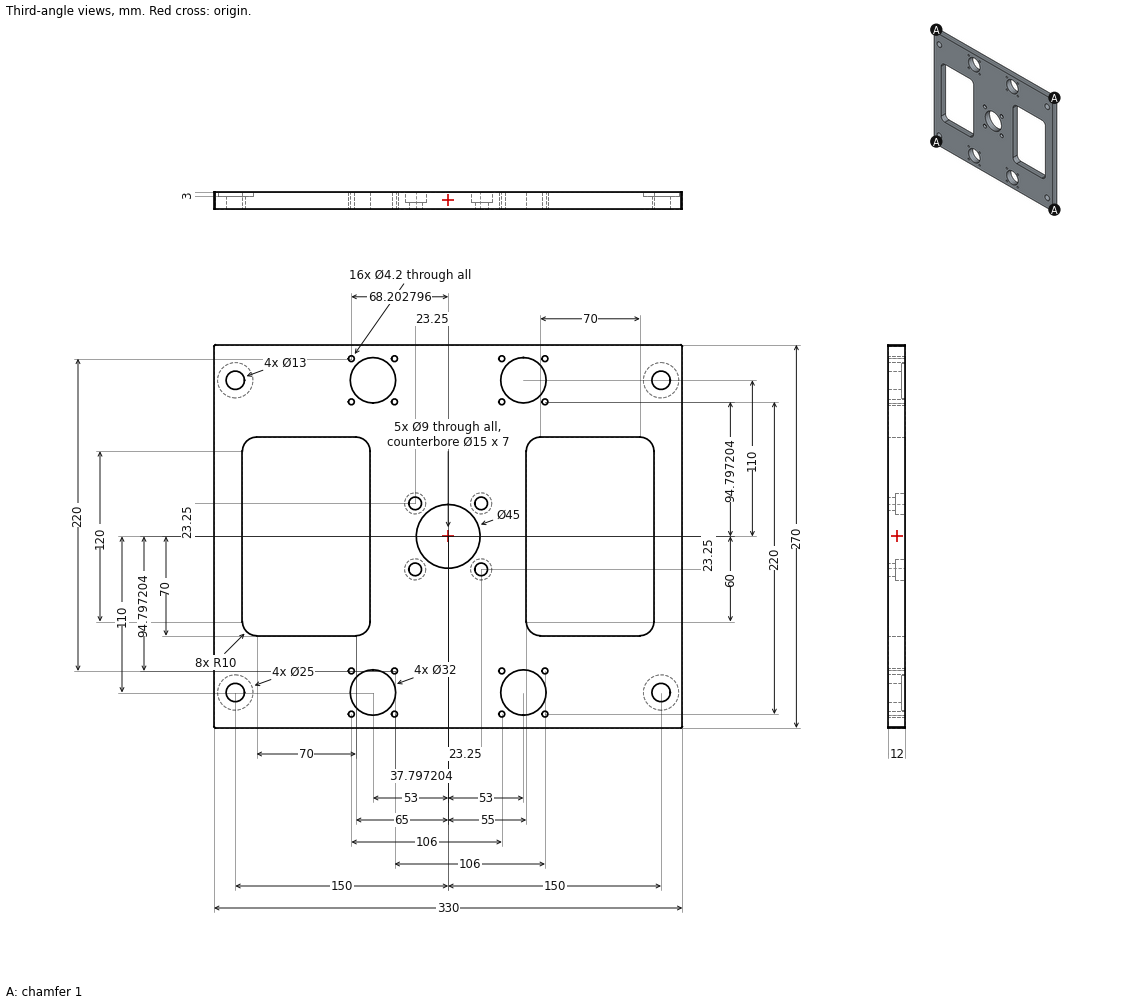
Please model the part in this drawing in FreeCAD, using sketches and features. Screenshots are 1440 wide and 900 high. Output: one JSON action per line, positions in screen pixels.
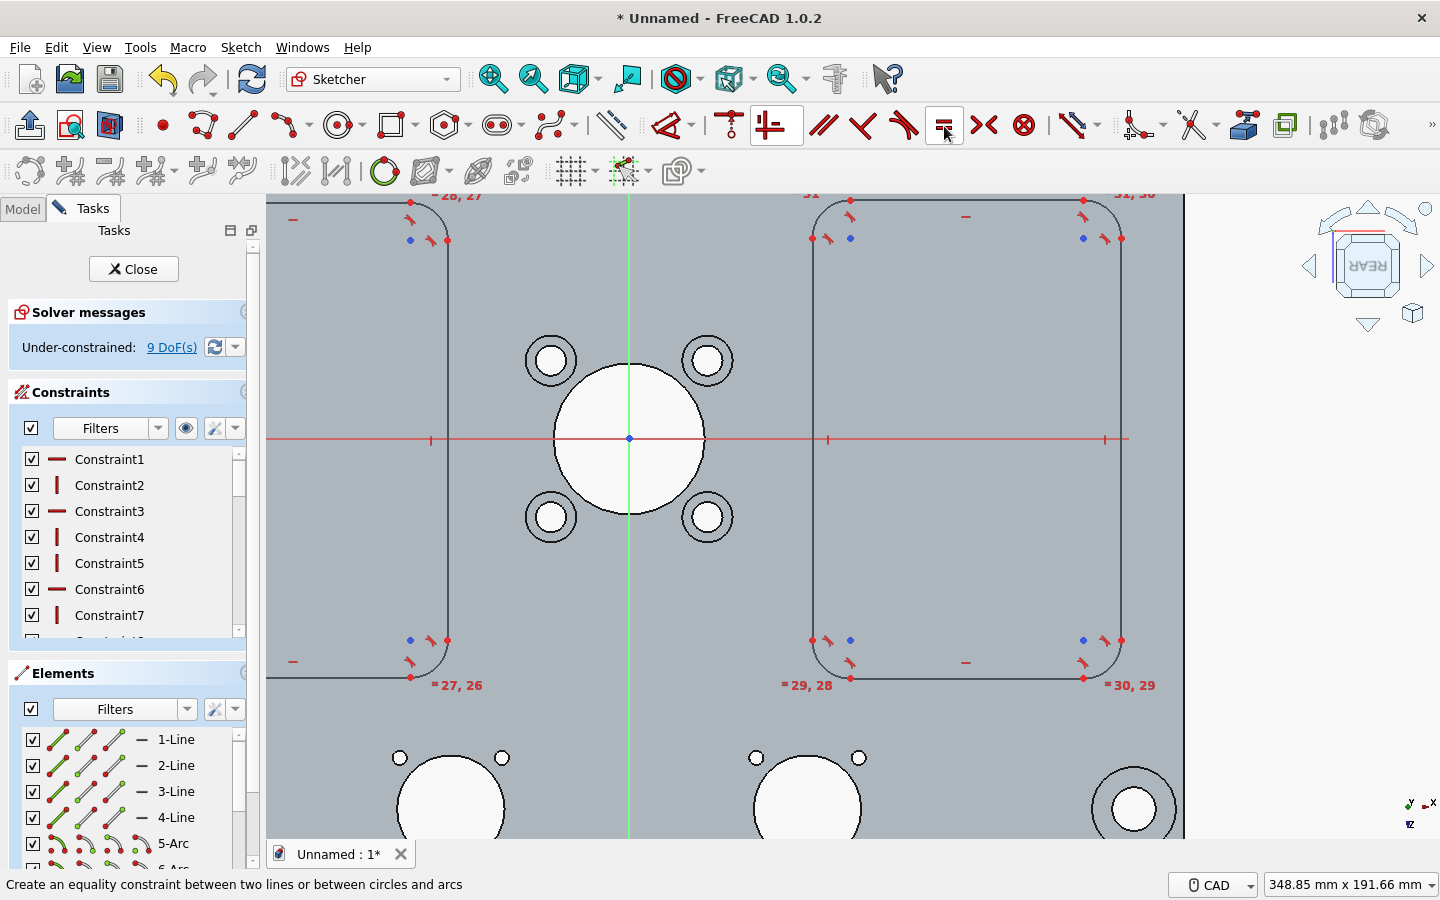
{"action": "scroll", "coordinate": [1100, 674], "scroll_direction": "down", "scroll_amount": 2}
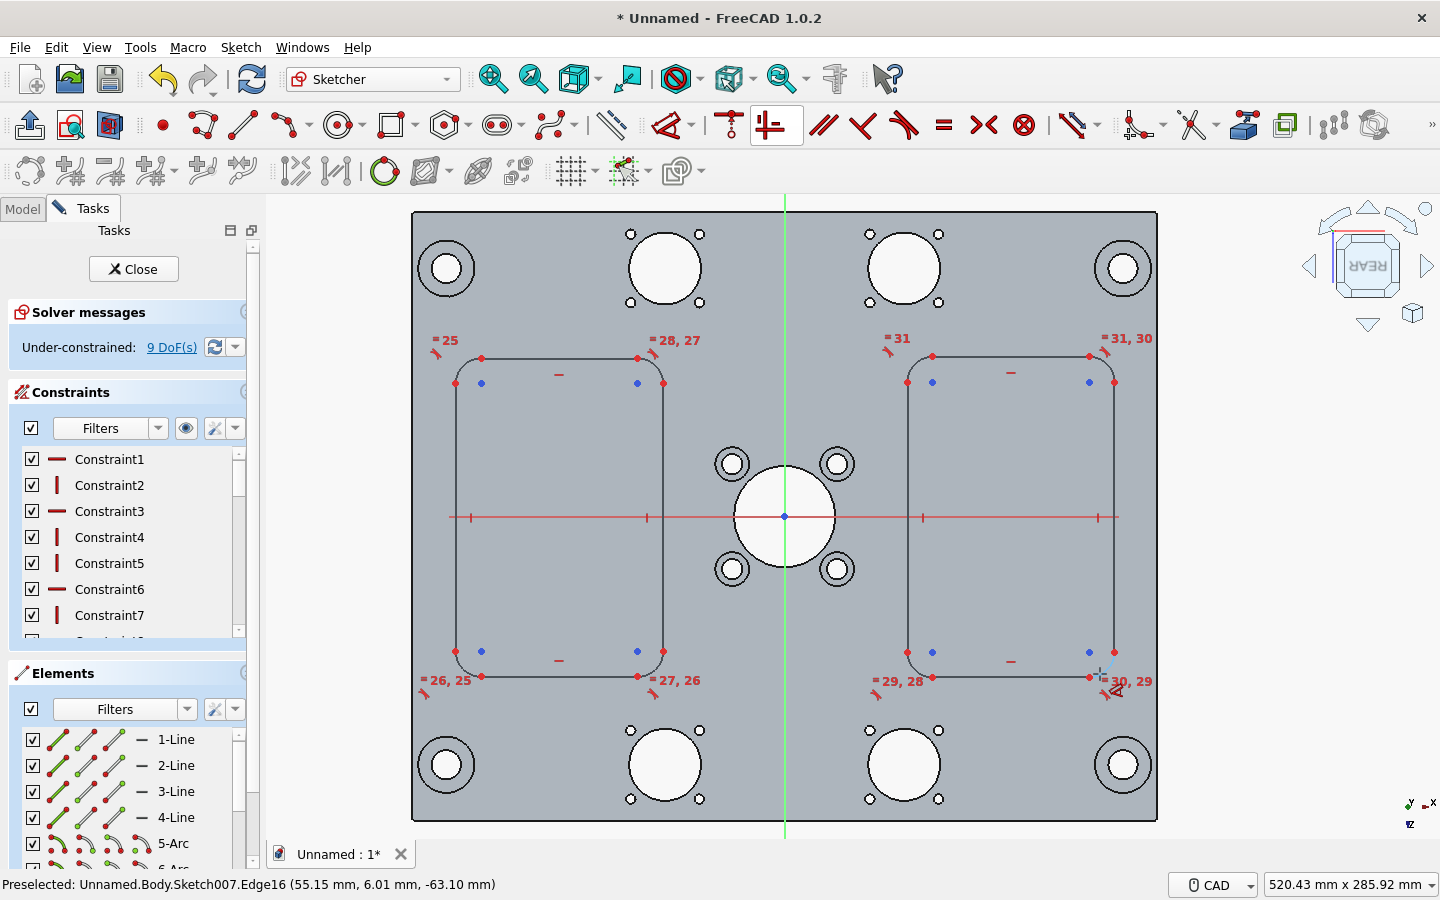
{"action": "scroll", "coordinate": [470, 361], "scroll_direction": "up", "scroll_amount": 3}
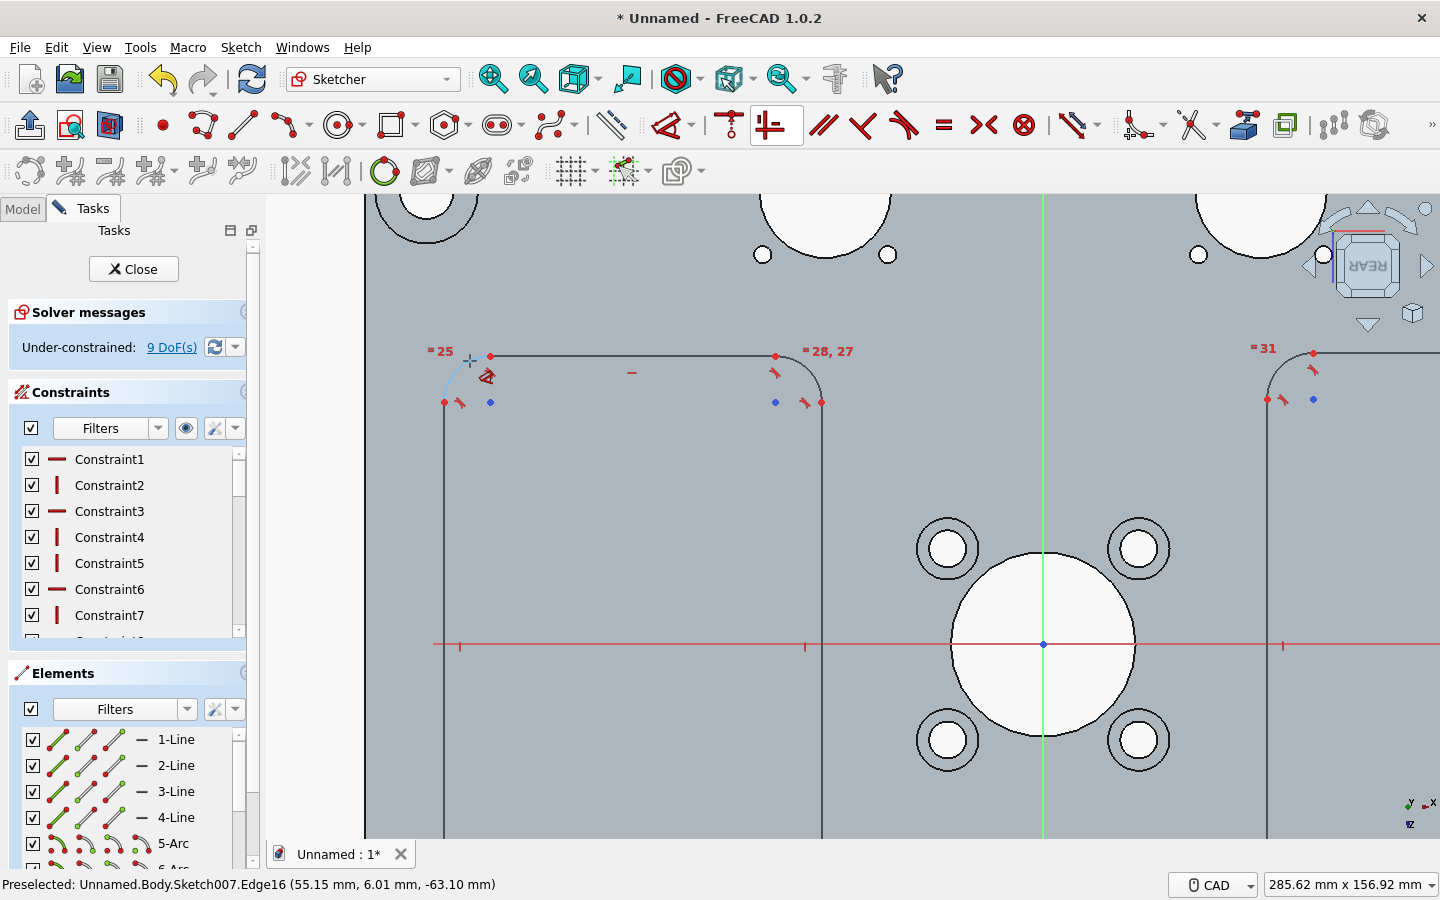
{"action": "left_click", "coordinate": [469, 361]}
{"action": "left_click", "coordinate": [454, 332]}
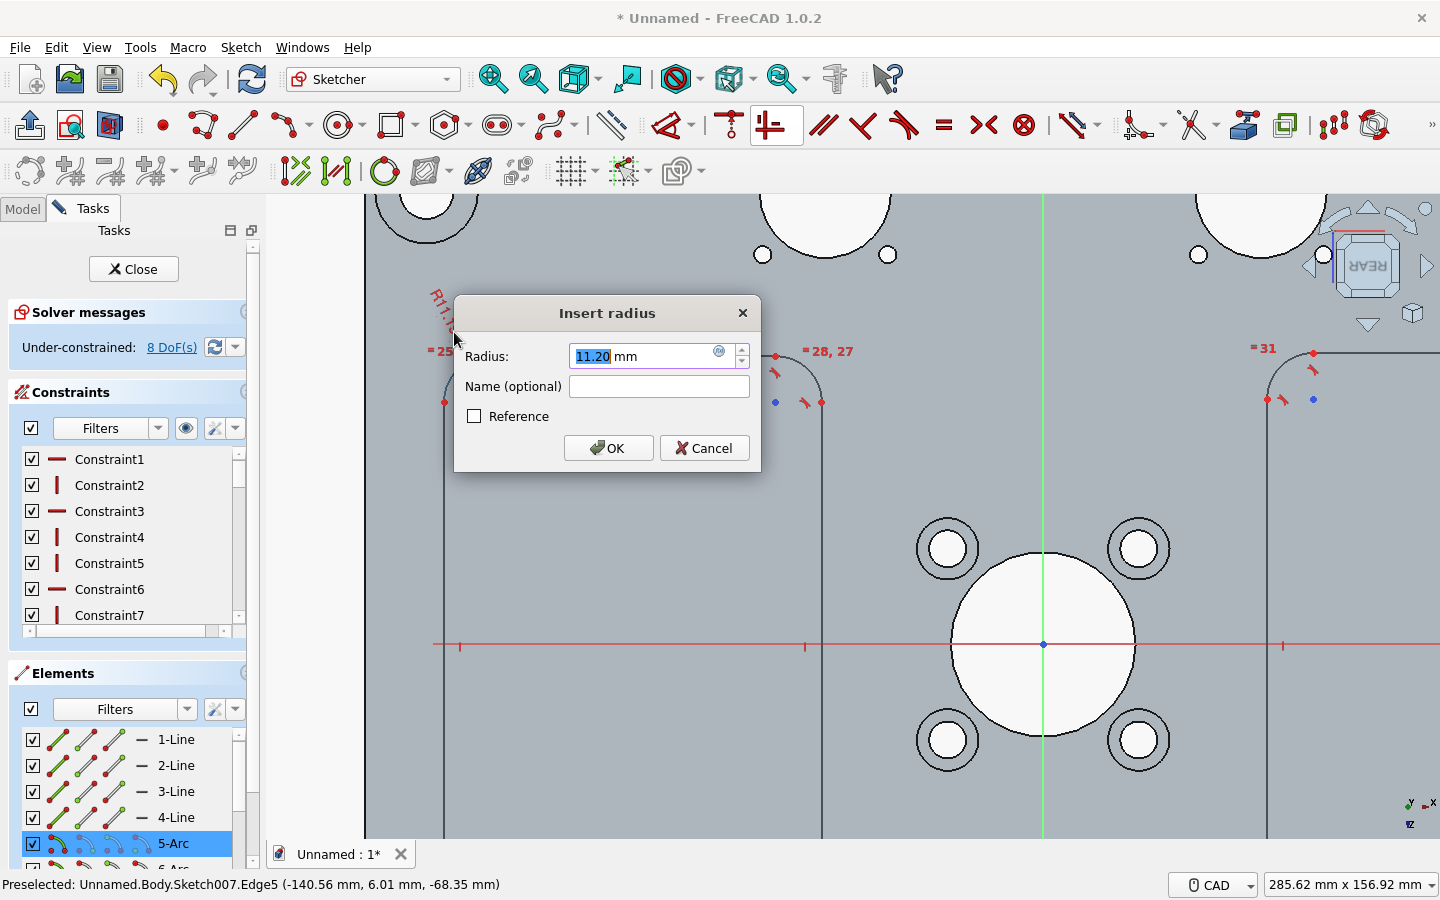
{"action": "type", "text": "10"}
{"action": "key", "text": "Return"}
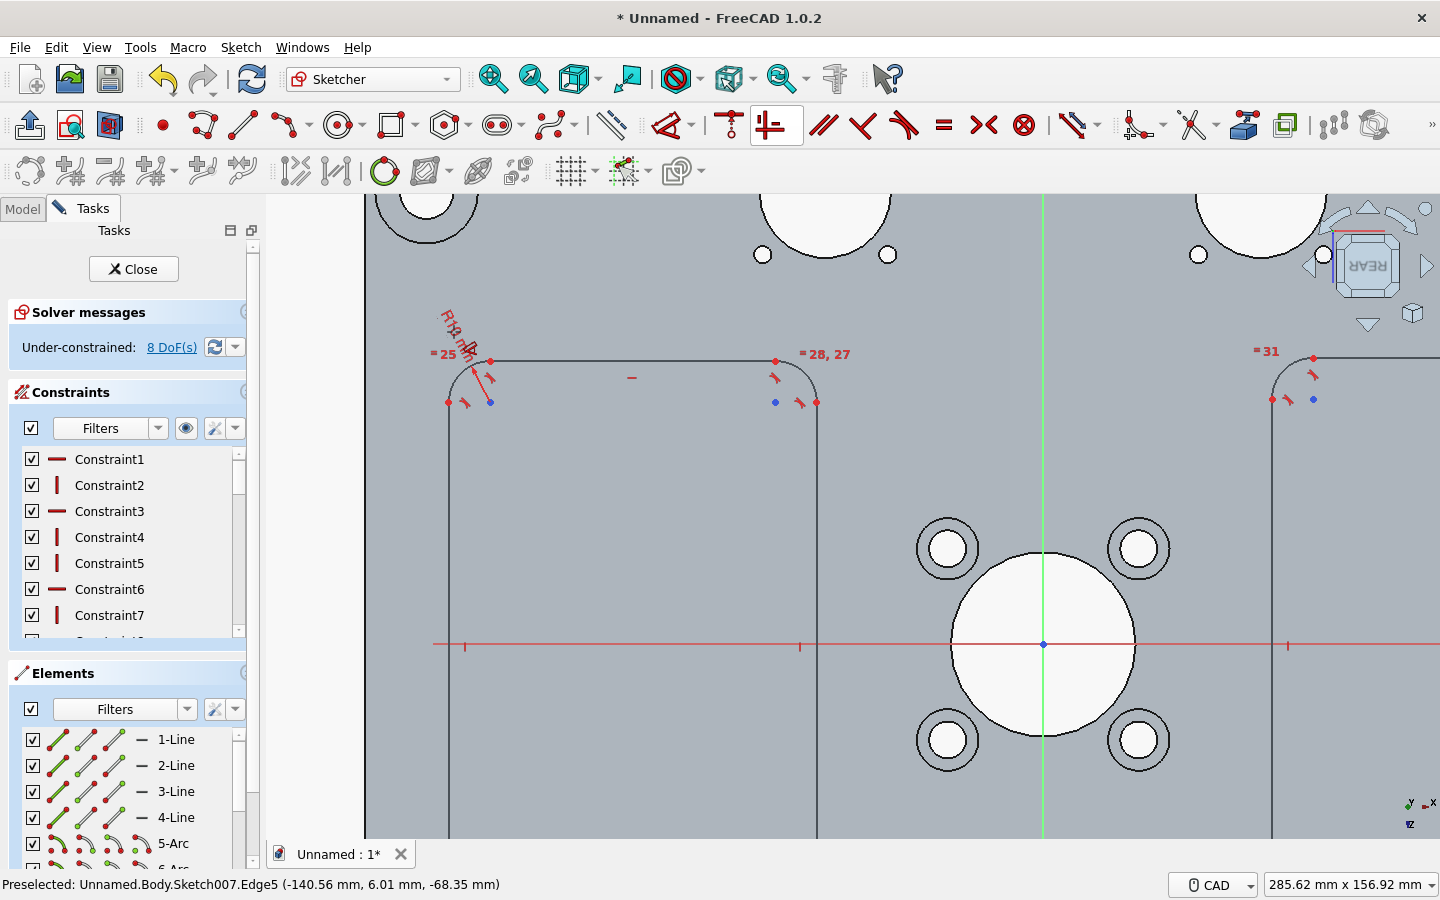
{"action": "left_click", "coordinate": [690, 361]}
{"action": "left_click", "coordinate": [633, 327]}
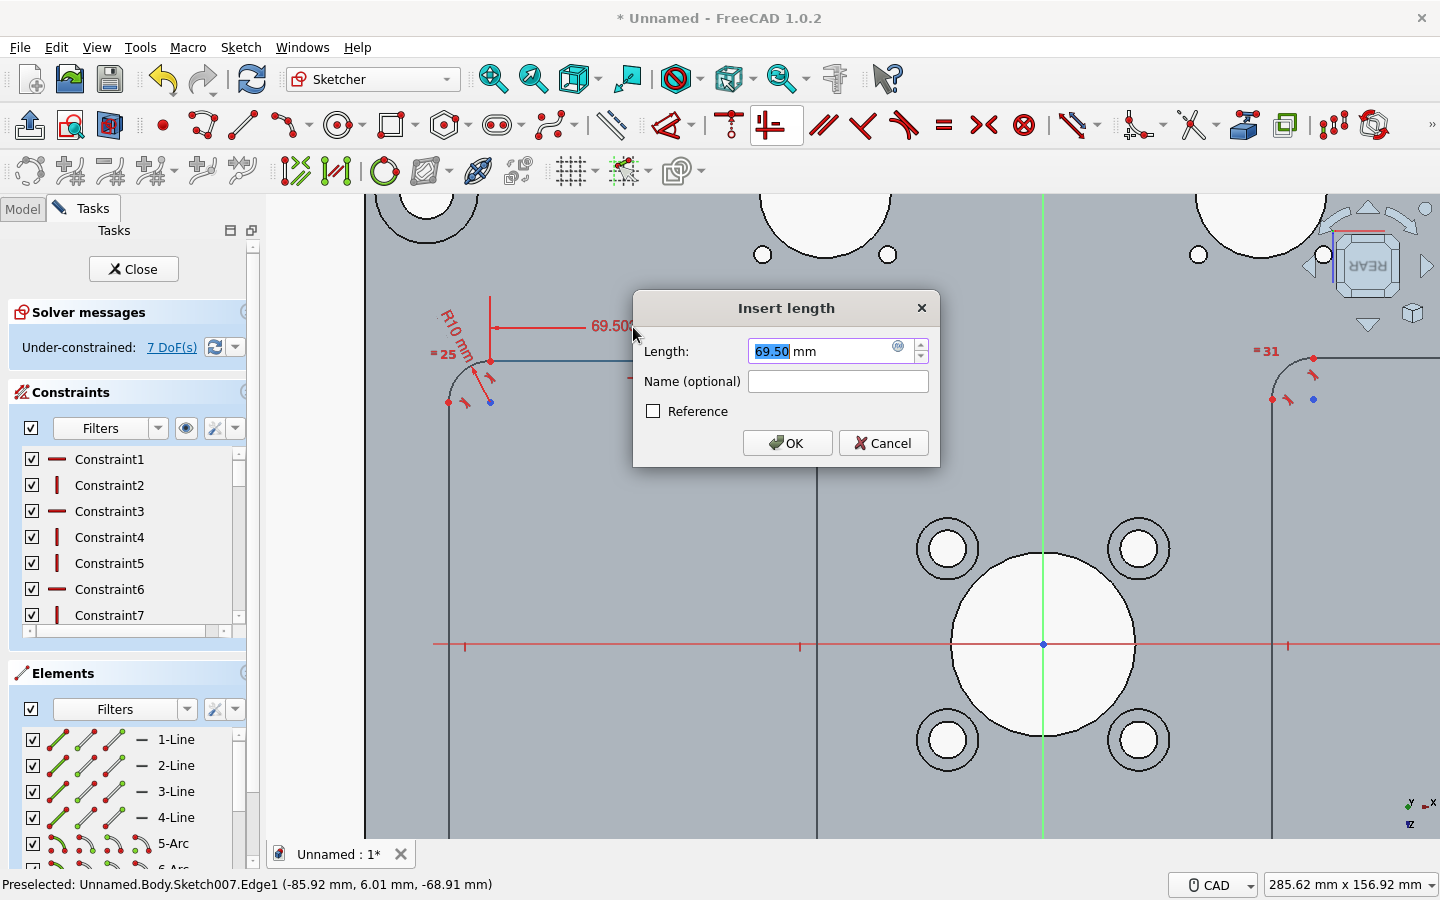
{"action": "type", "text": "70"}
{"action": "key", "text": "Return"}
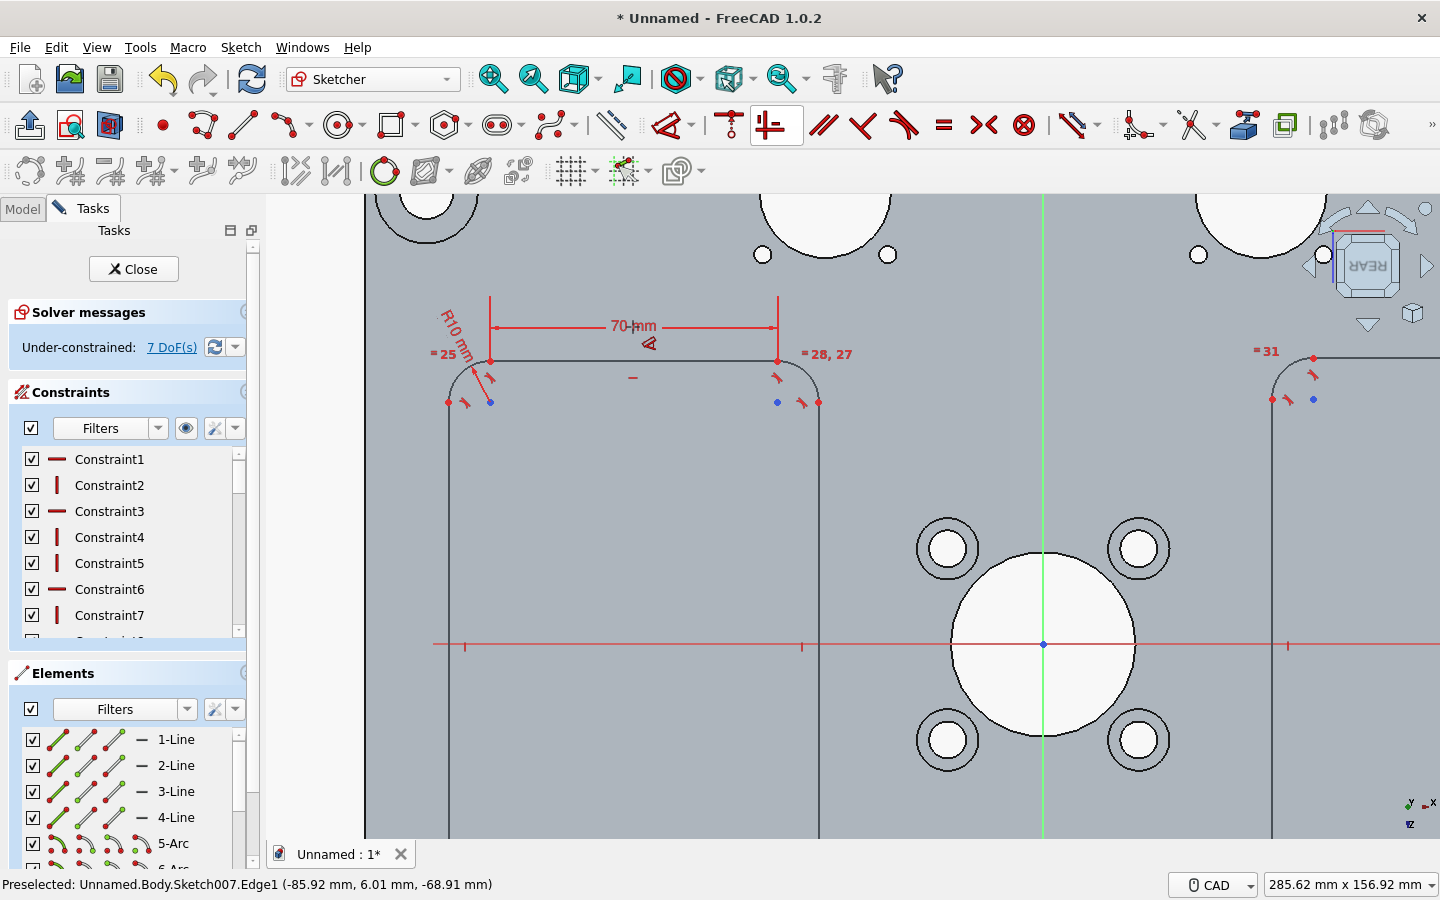
{"action": "scroll", "coordinate": [470, 361], "scroll_direction": "down", "scroll_amount": 3}